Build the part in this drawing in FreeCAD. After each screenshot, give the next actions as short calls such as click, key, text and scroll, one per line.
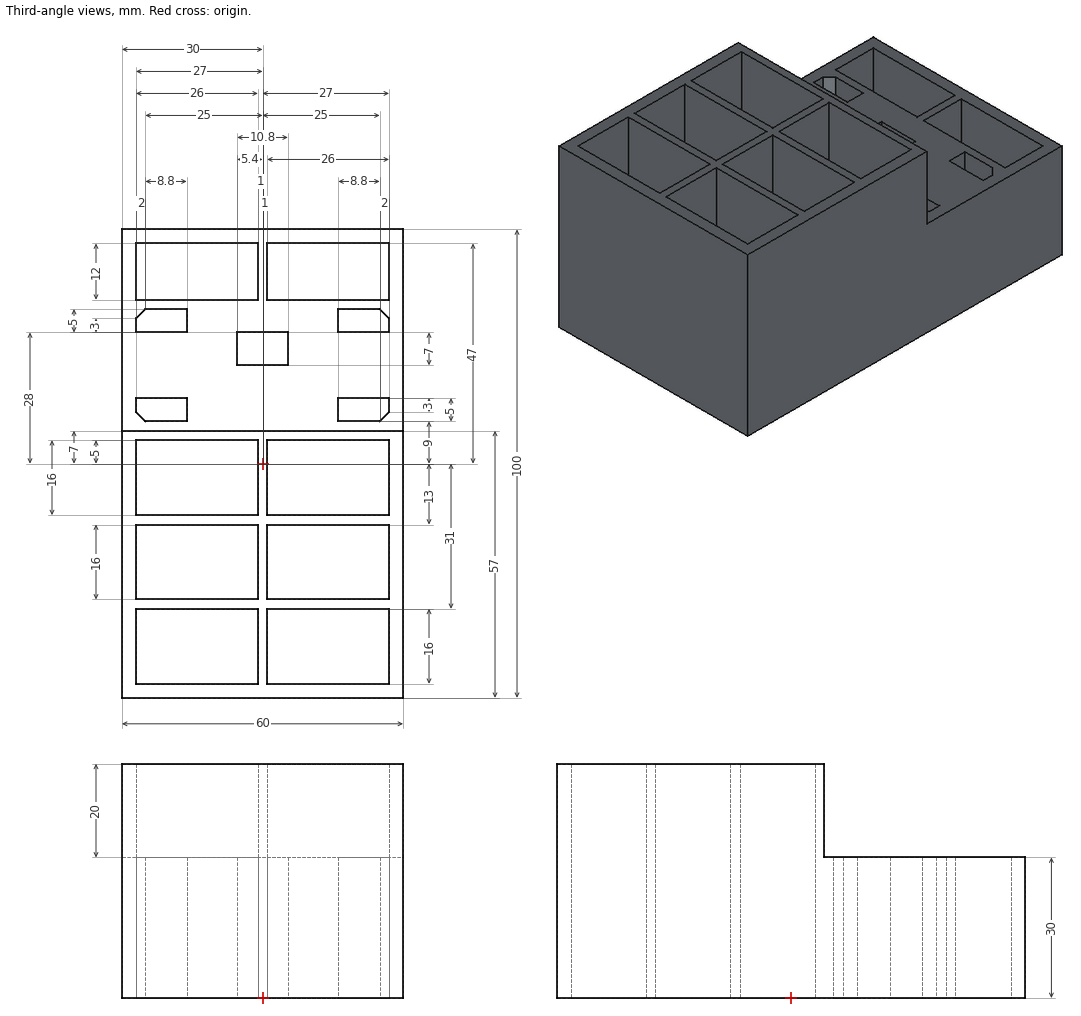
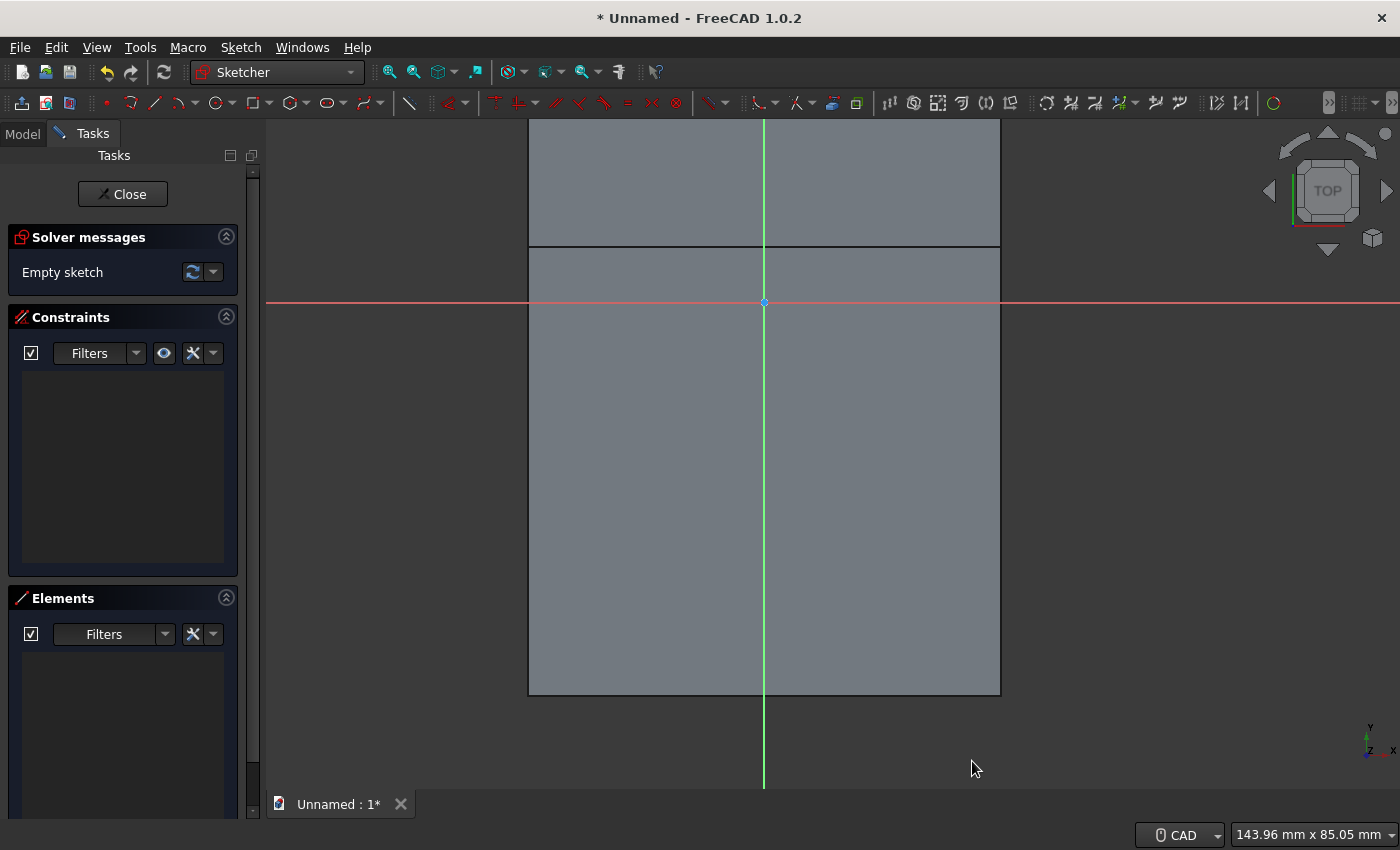
key(g)
key(r)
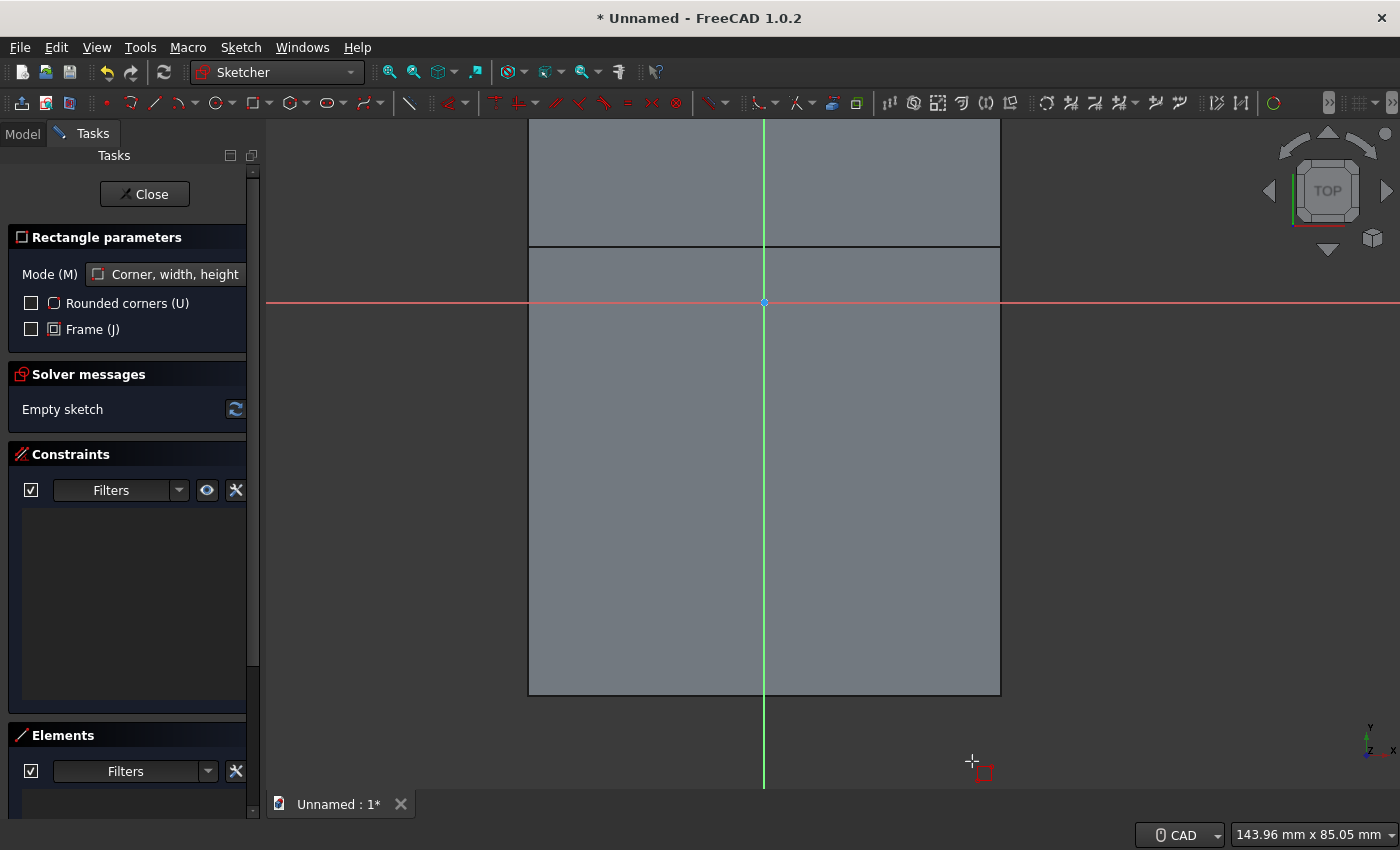
click(552, 263)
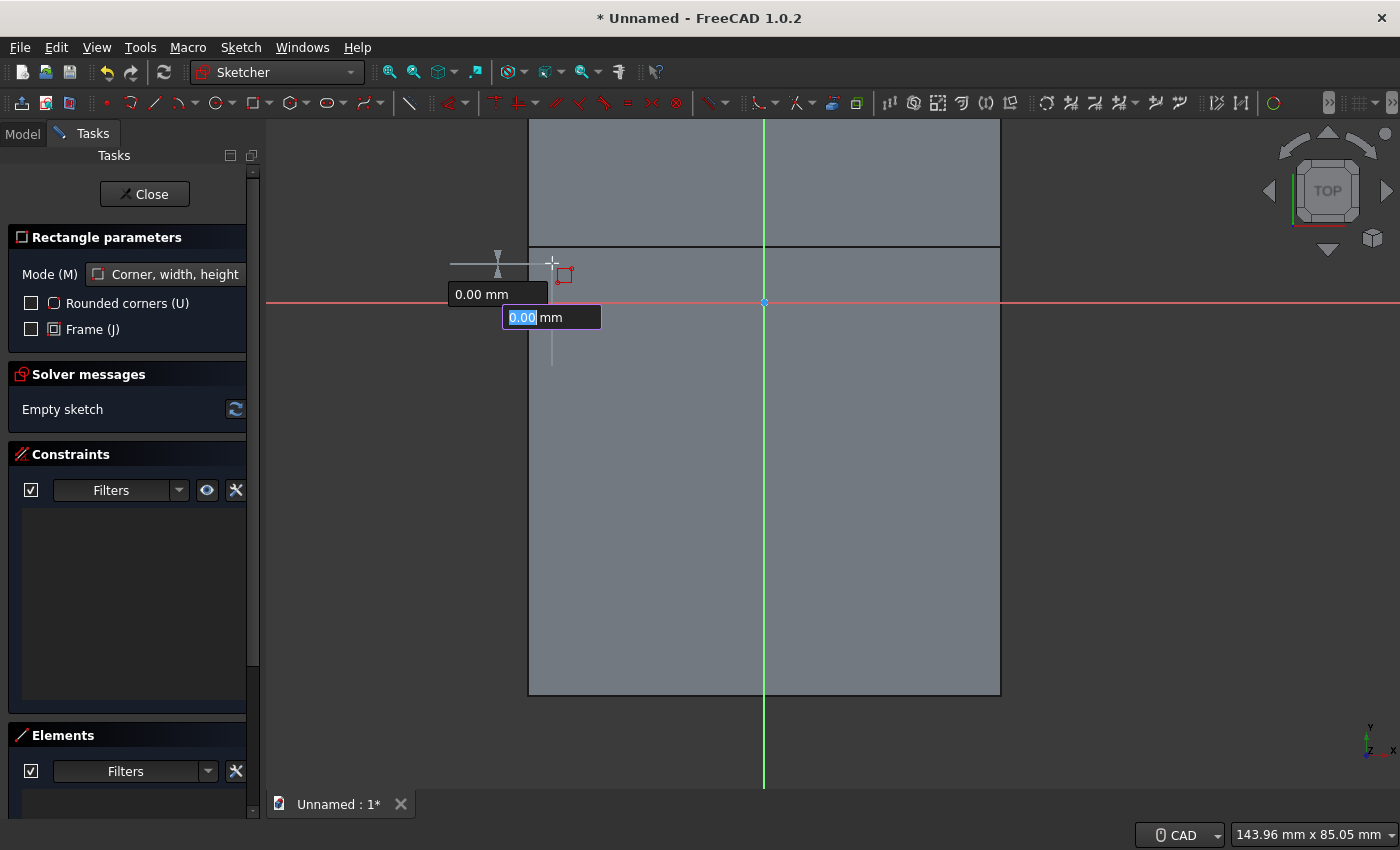
scroll(756, 389, up, 4)
move(756, 389)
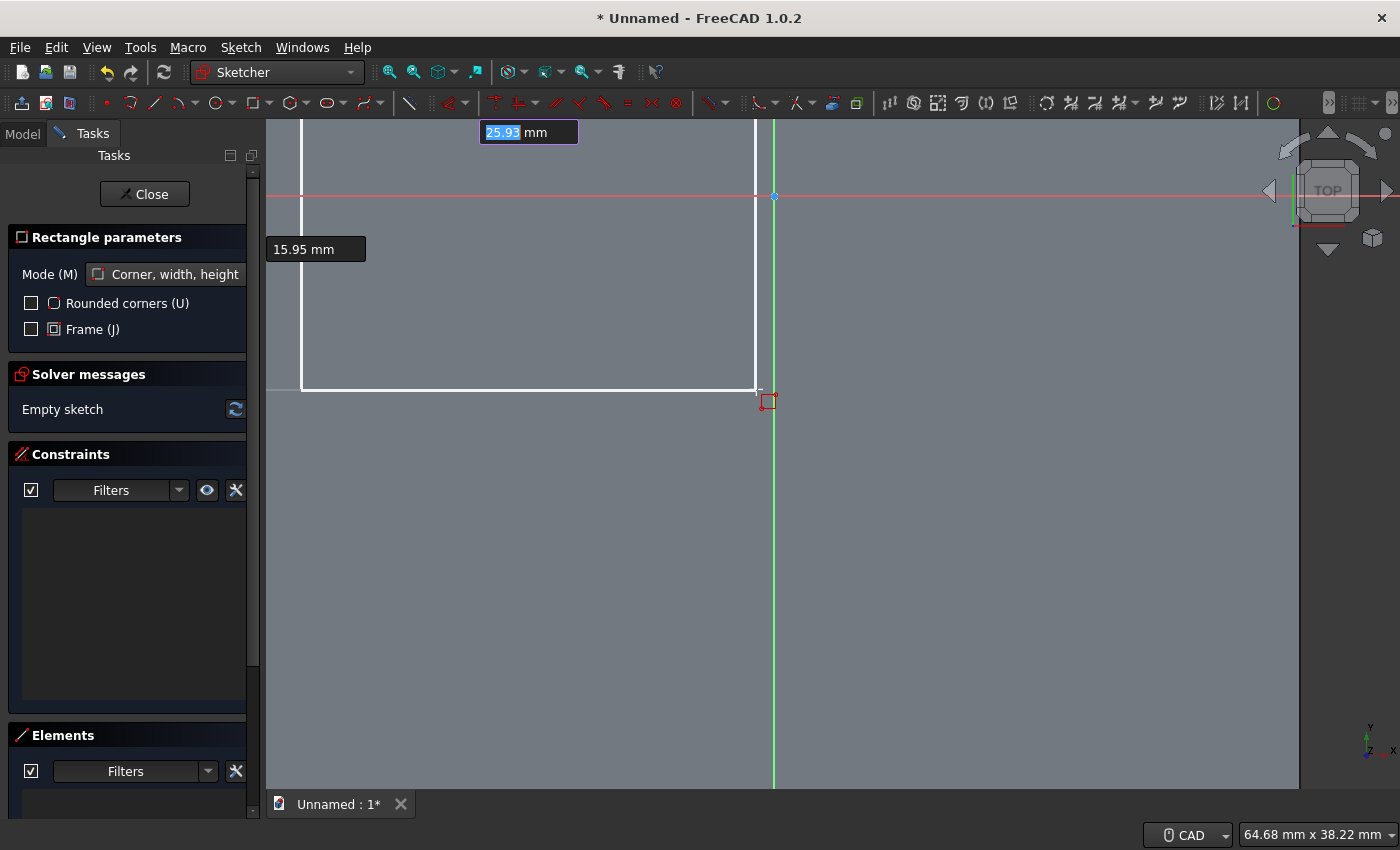
text(26)
key(Tab)
text(16)
key(Return)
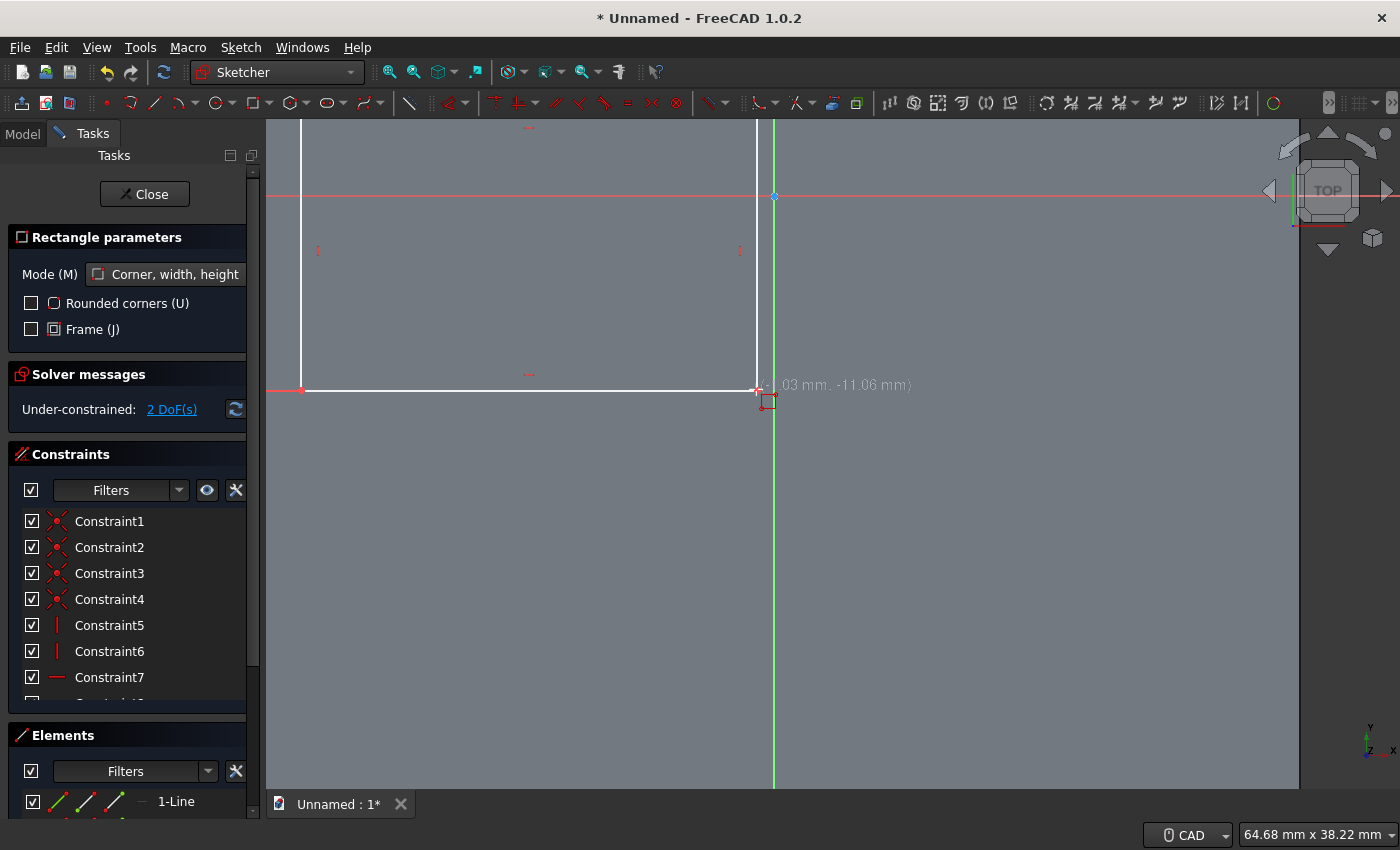
scroll(757, 364, down, 4)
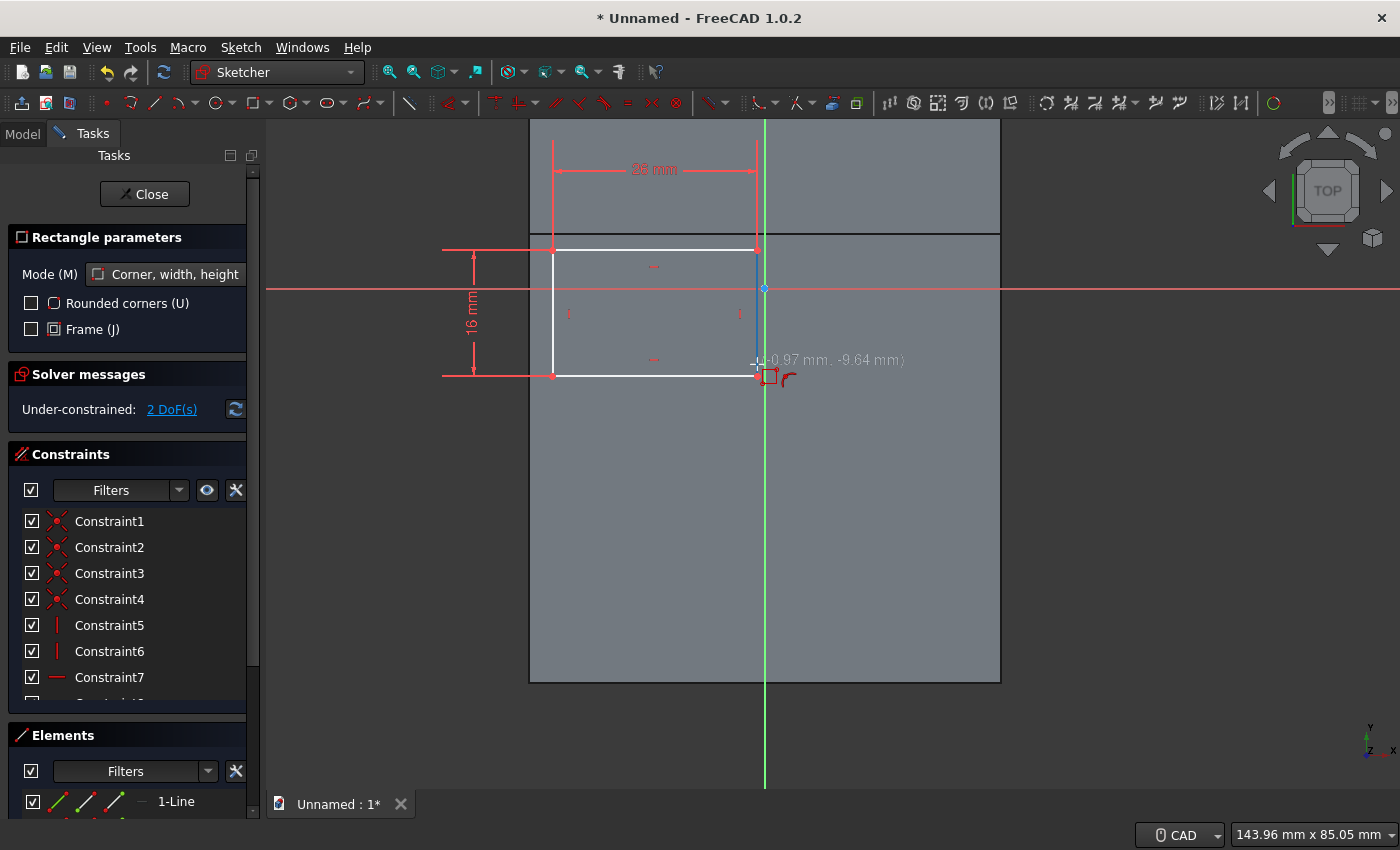
scroll(773, 249, up, 4)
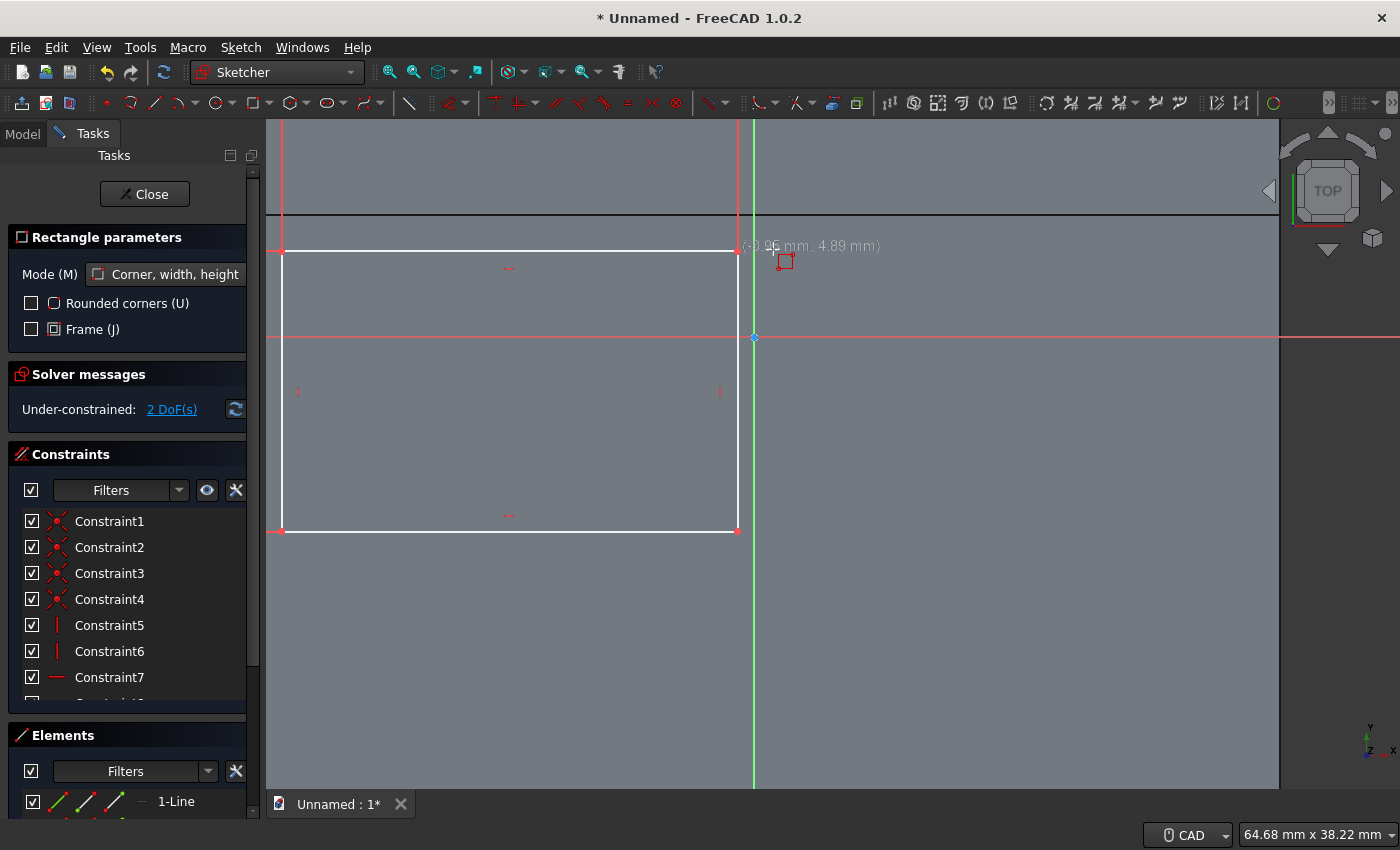
click(772, 250)
move(1228, 530)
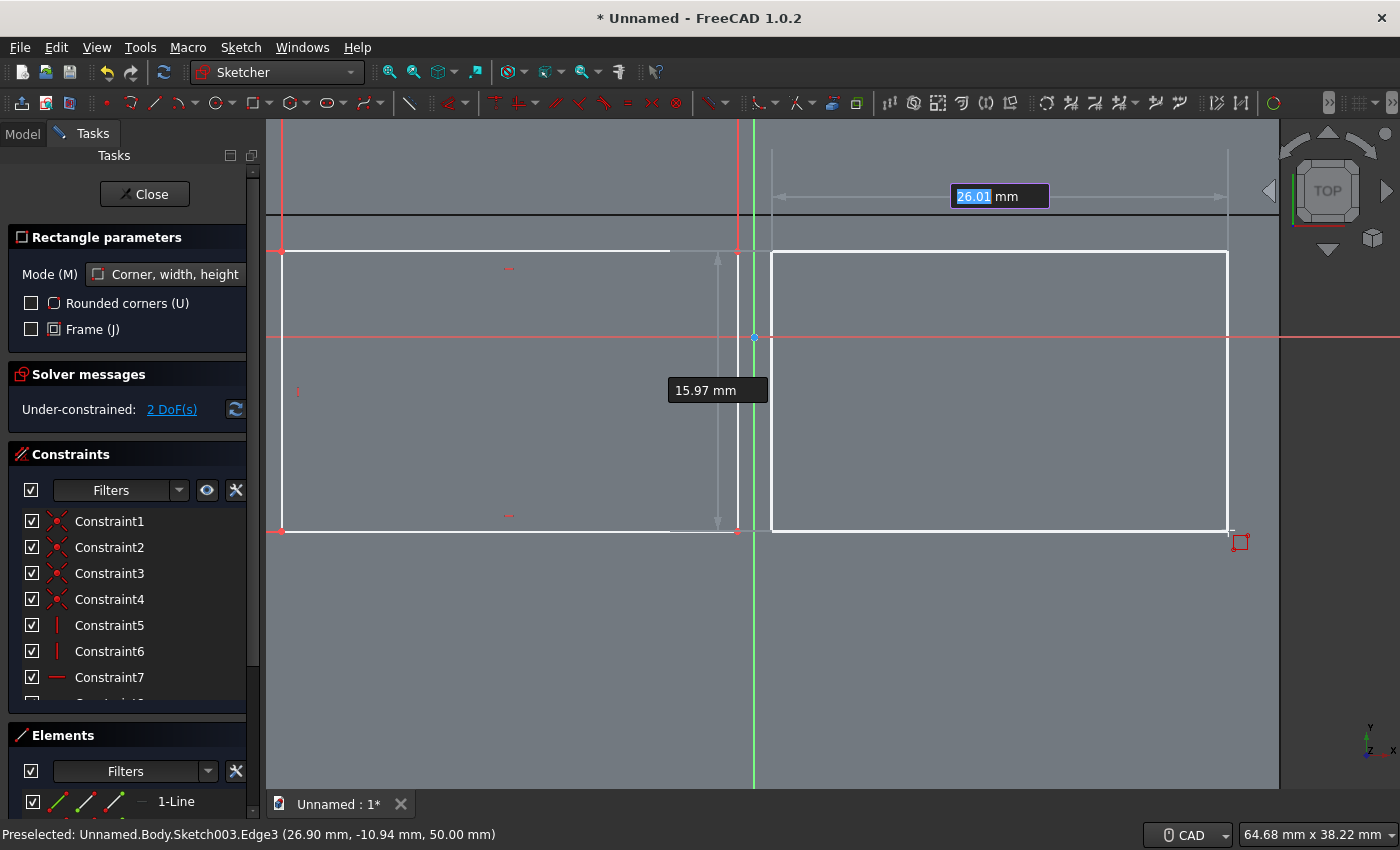
text(26)
key(Tab)
text(16)
key(Return)